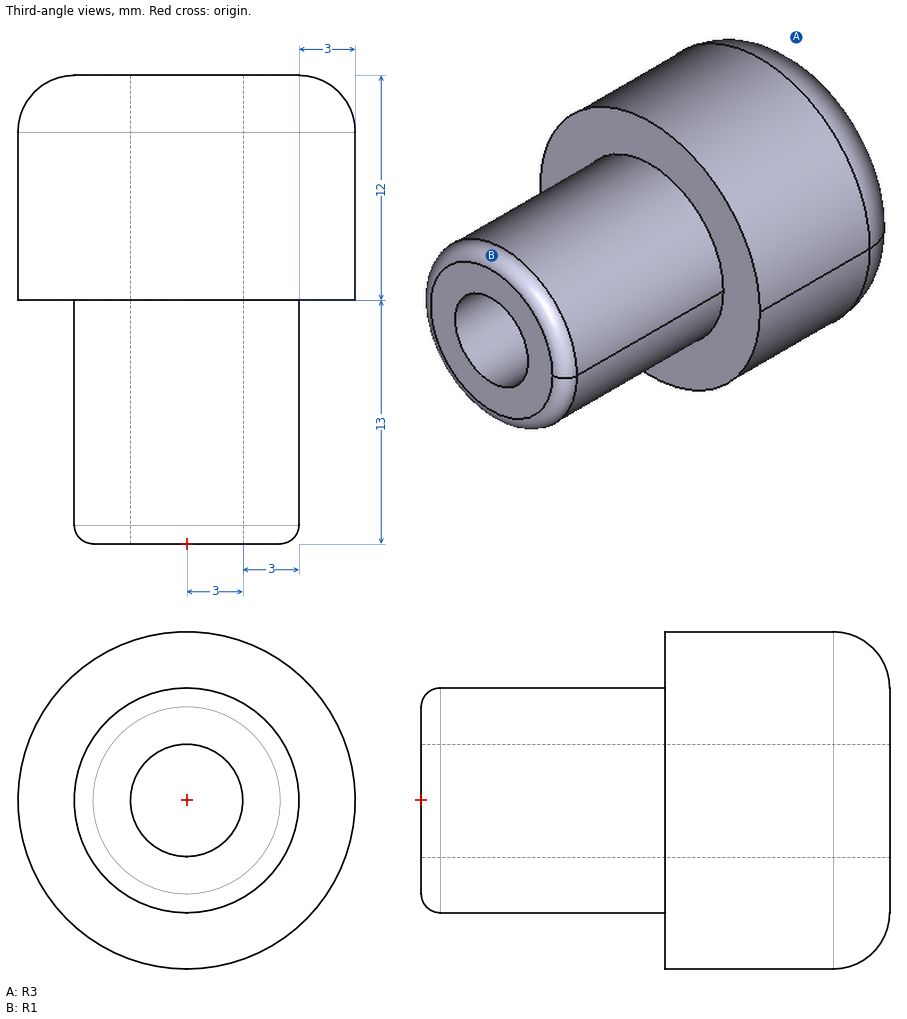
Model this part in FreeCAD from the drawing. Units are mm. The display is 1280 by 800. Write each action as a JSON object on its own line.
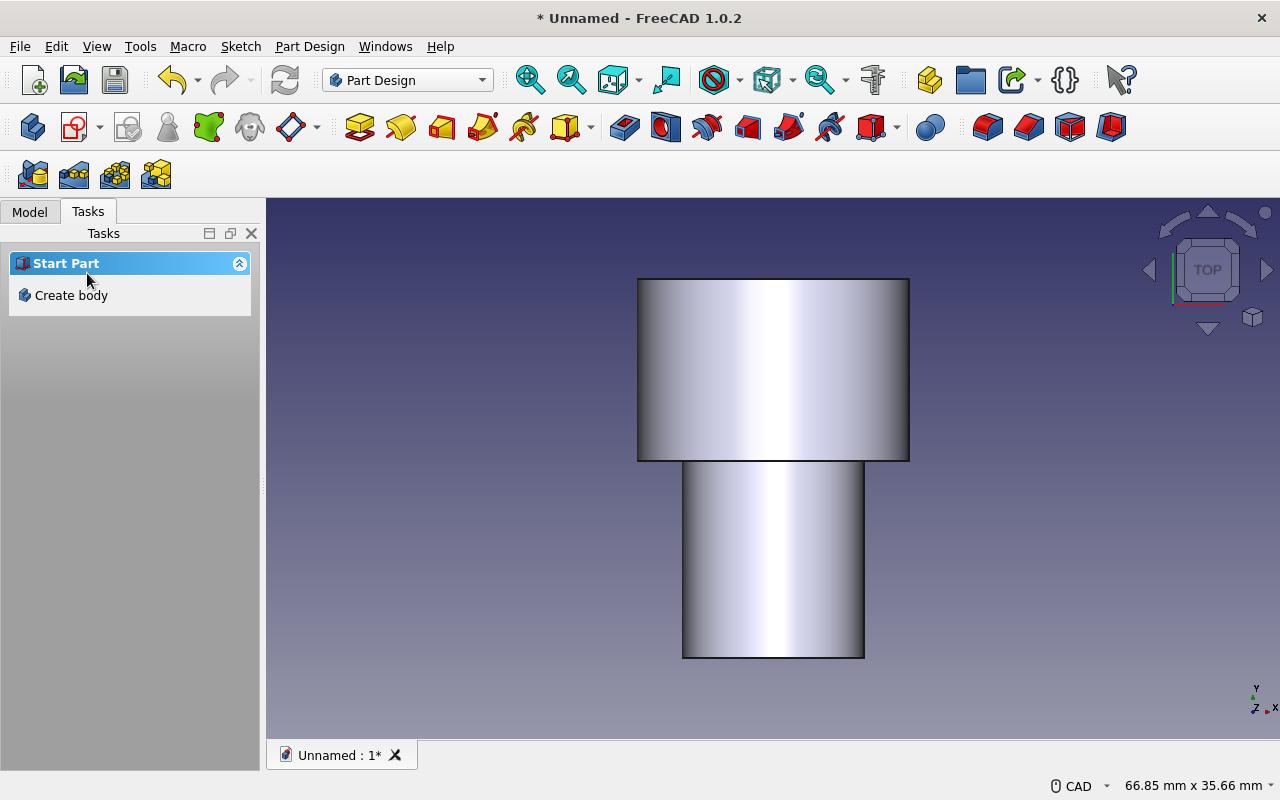
{"action": "left_click", "coordinate": [662, 278]}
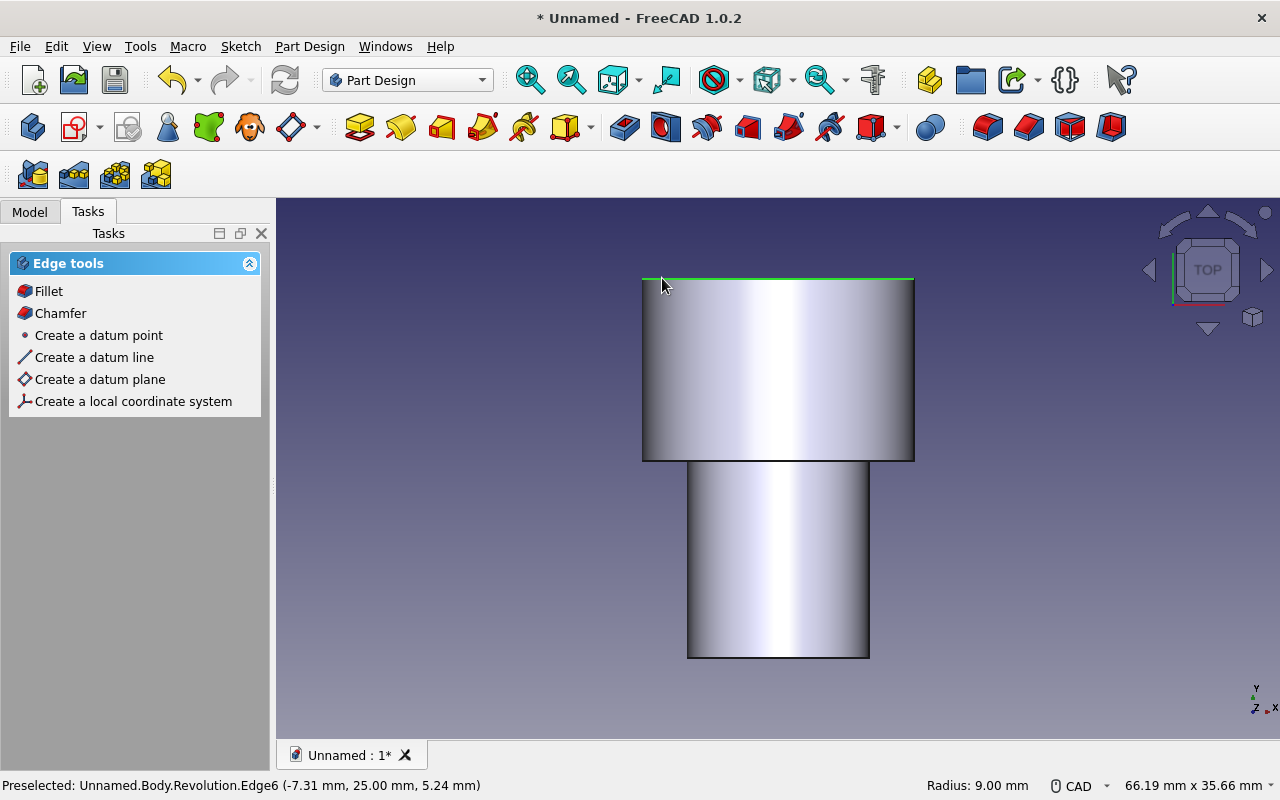
{"action": "left_click", "coordinate": [988, 128]}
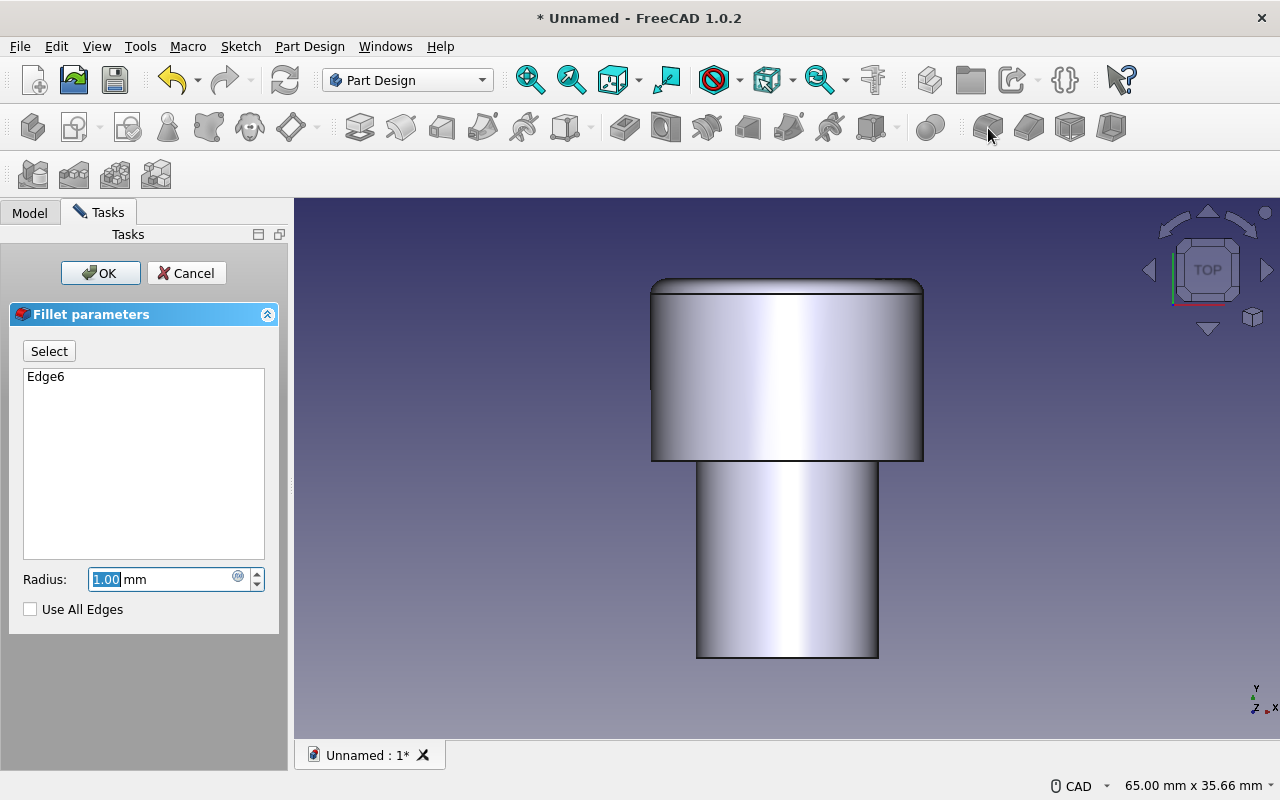
{"action": "type", "text": "3"}
{"action": "key", "text": "Tab"}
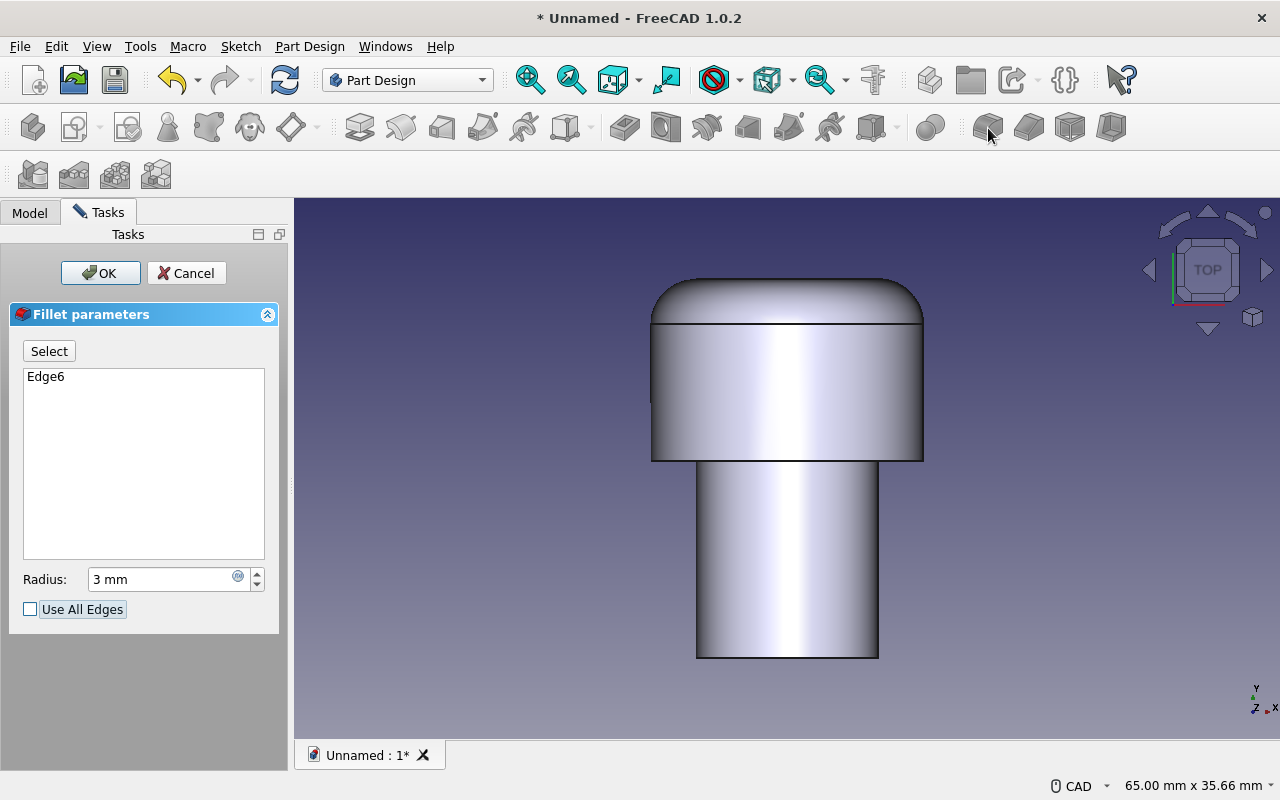
{"action": "left_click", "coordinate": [101, 273]}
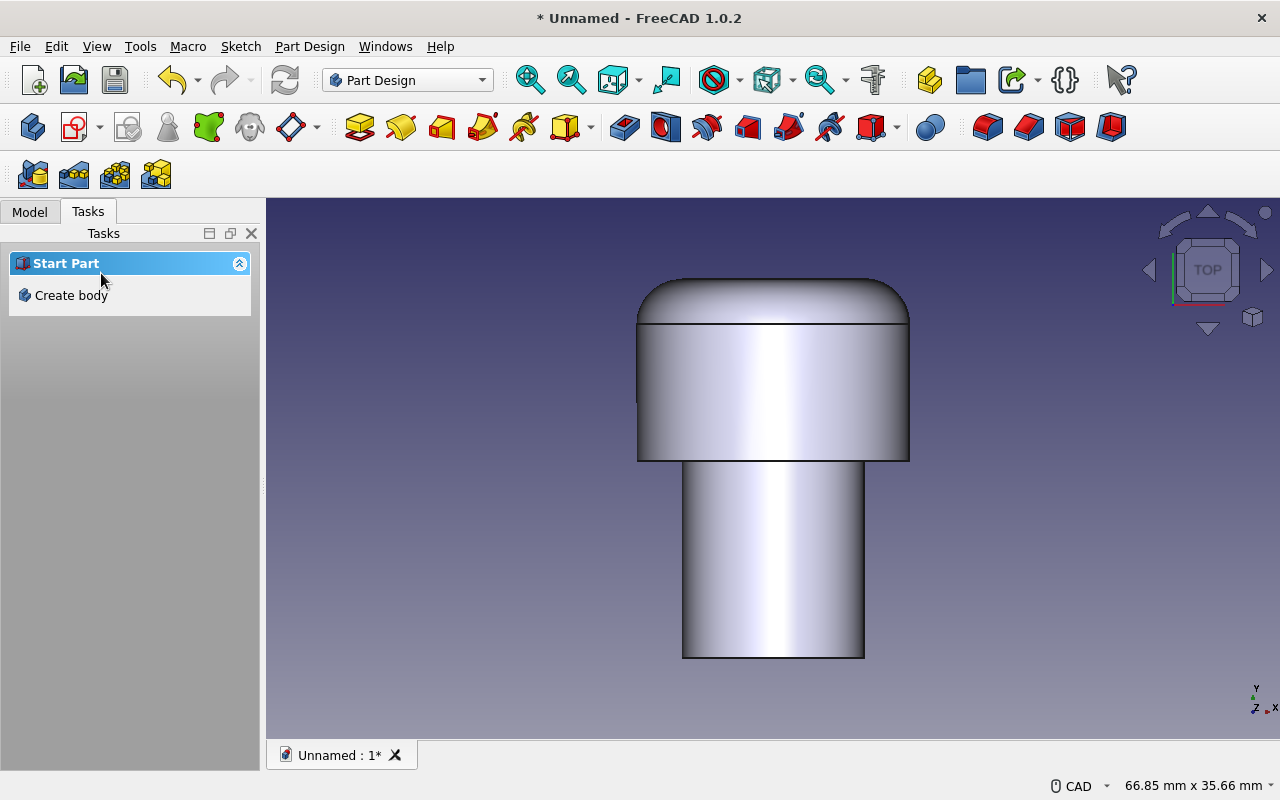
{"action": "left_click", "coordinate": [699, 657]}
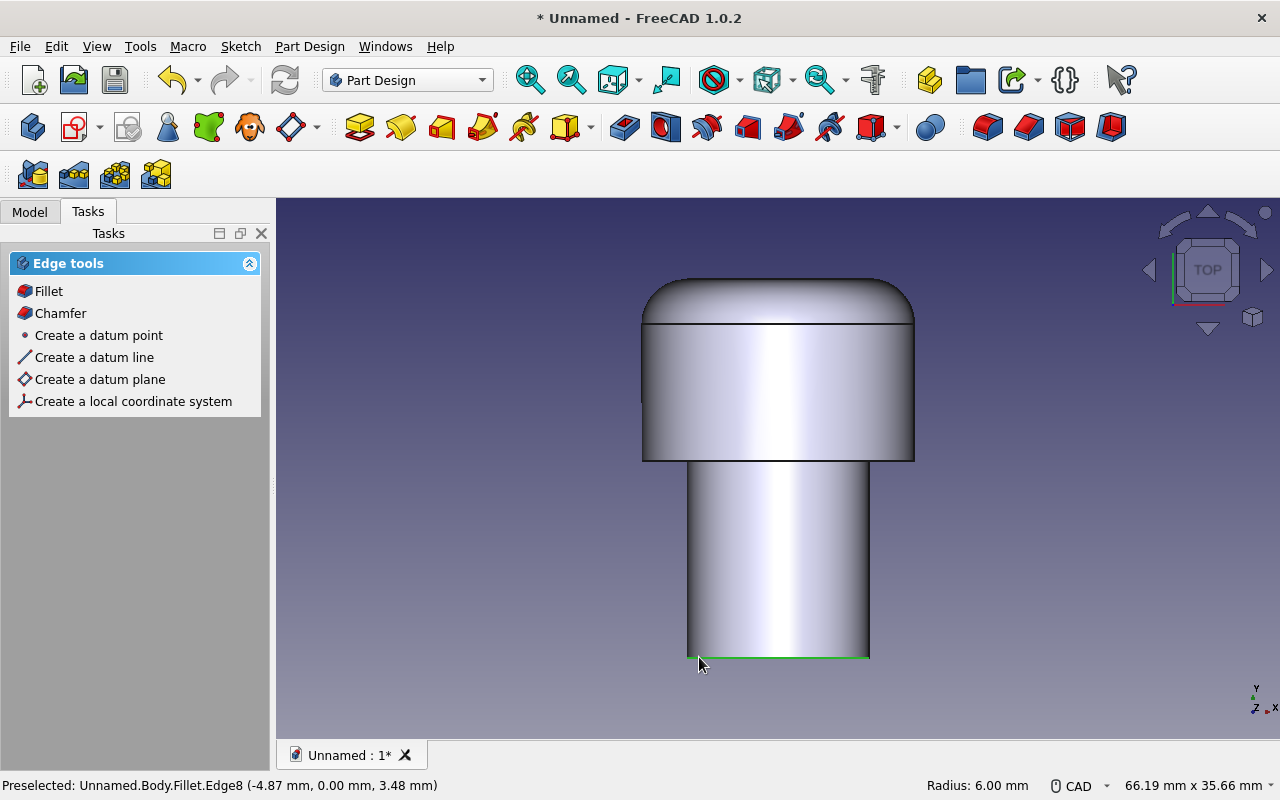
{"action": "left_click", "coordinate": [988, 128]}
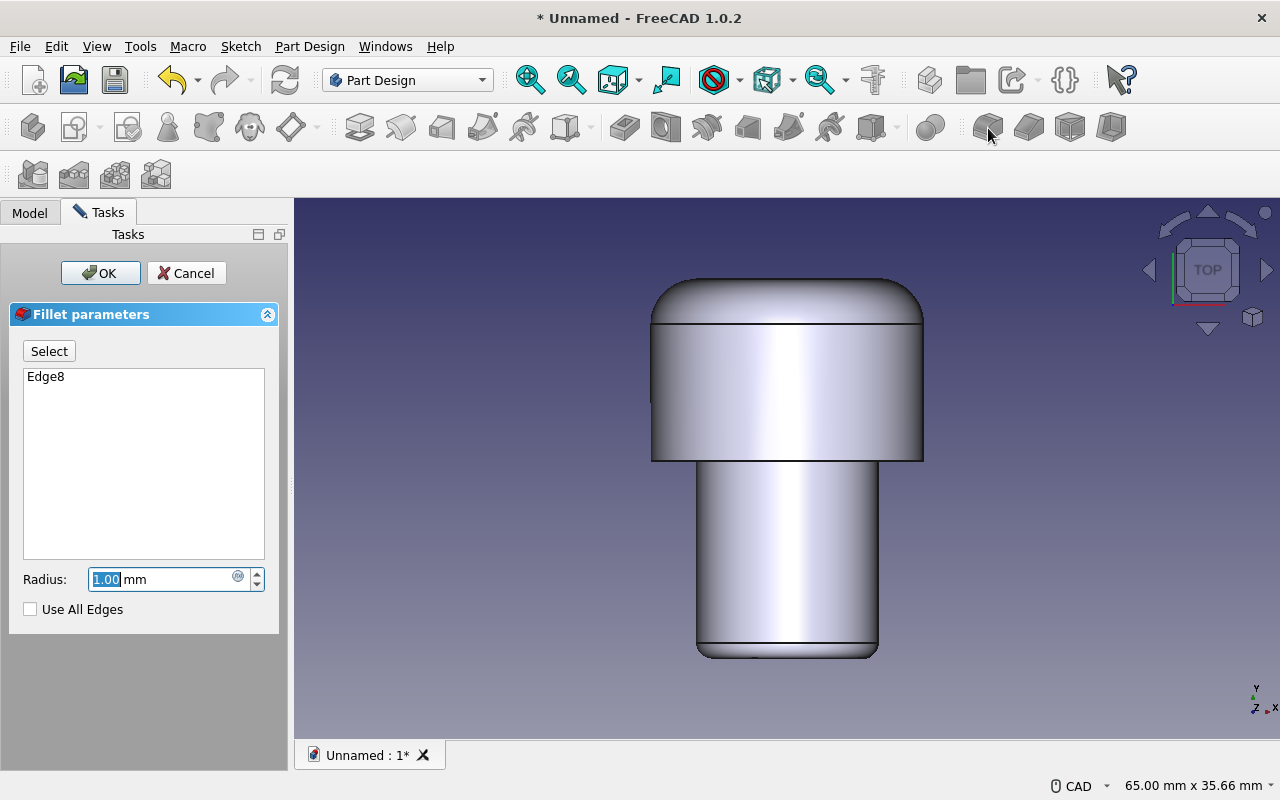
{"action": "type", "text": "1"}
{"action": "key", "text": "Tab"}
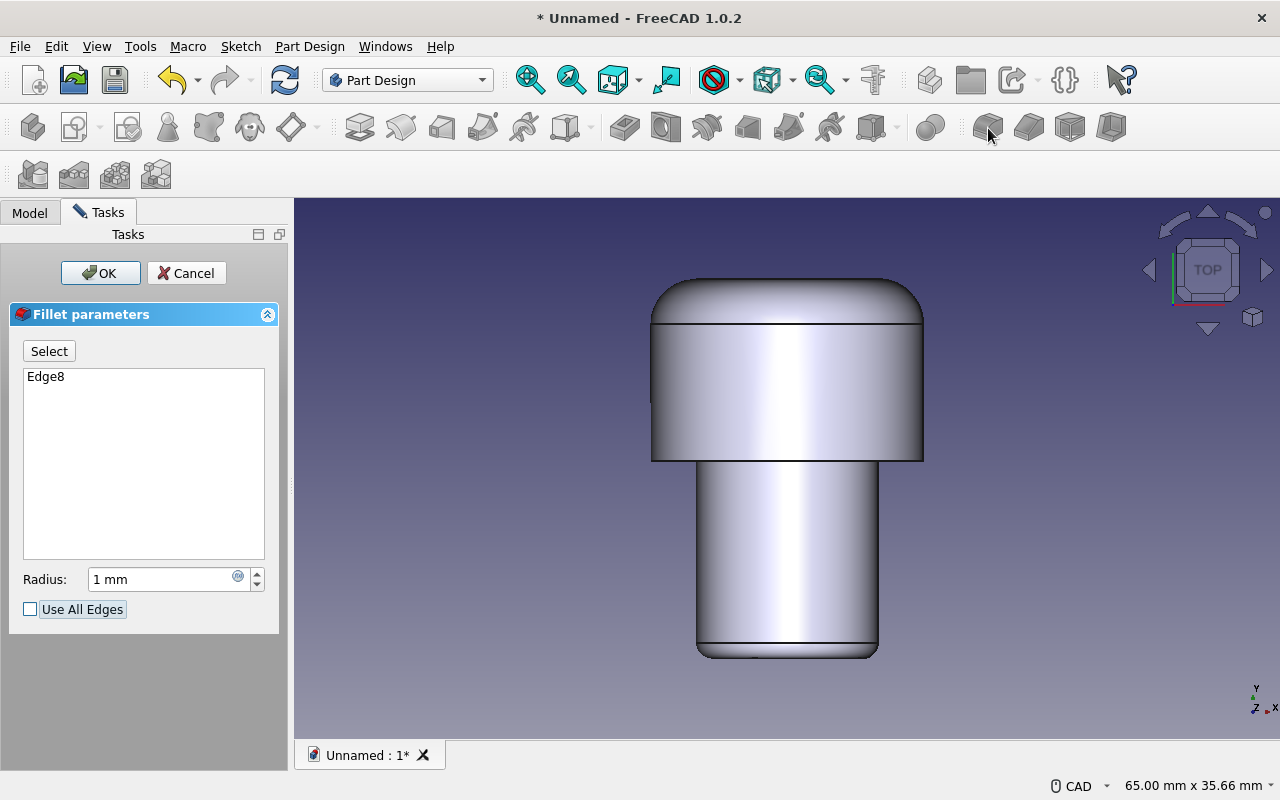
{"action": "left_click", "coordinate": [101, 273]}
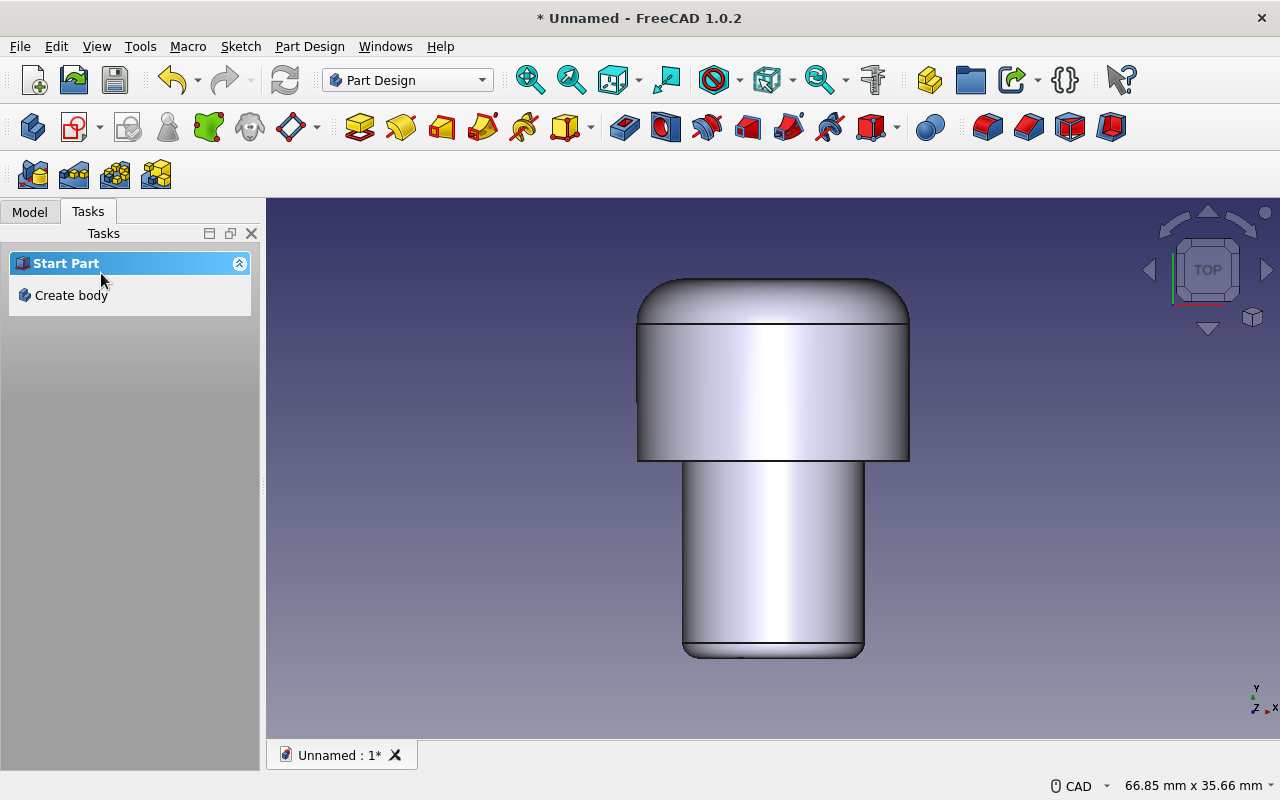
{"action": "key", "text": "0"}